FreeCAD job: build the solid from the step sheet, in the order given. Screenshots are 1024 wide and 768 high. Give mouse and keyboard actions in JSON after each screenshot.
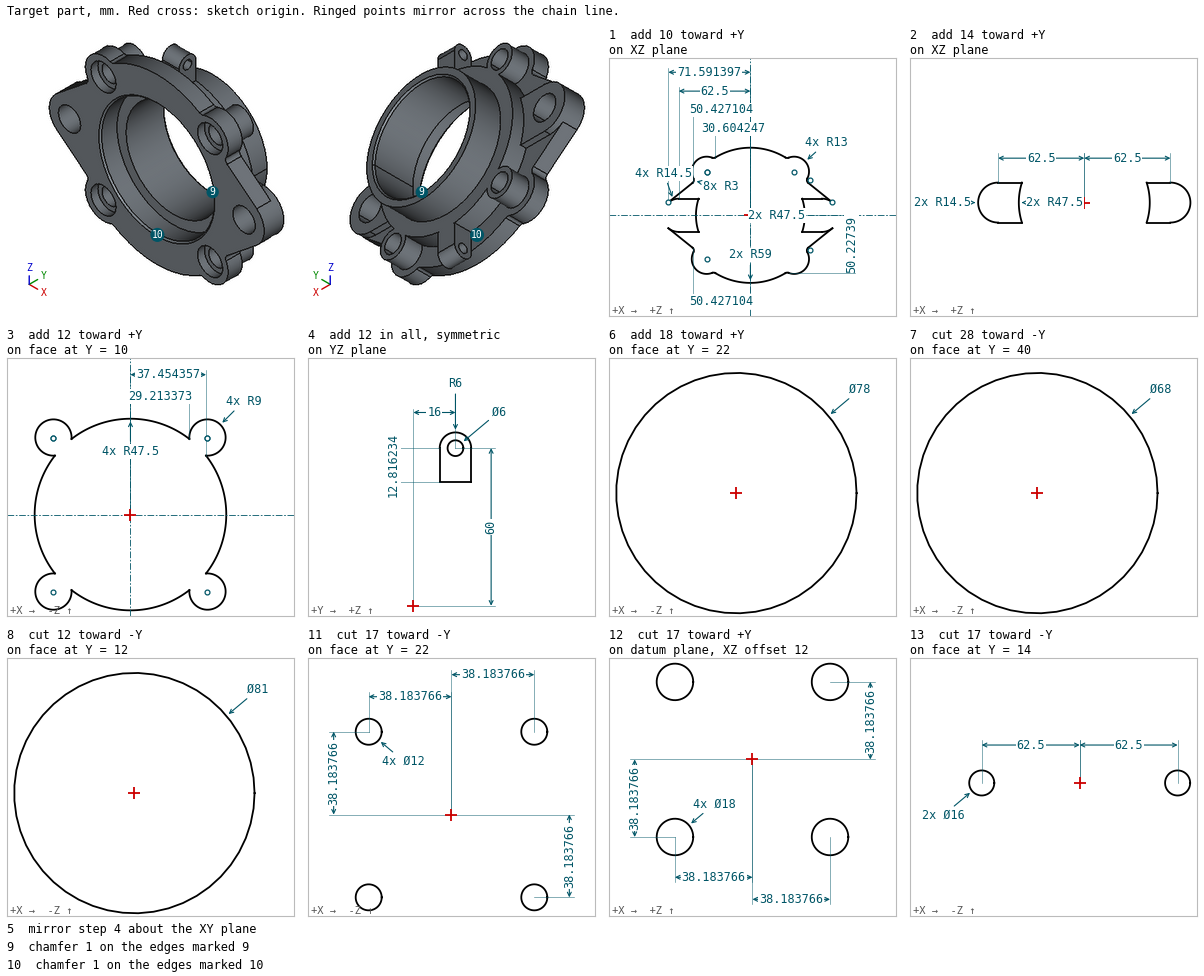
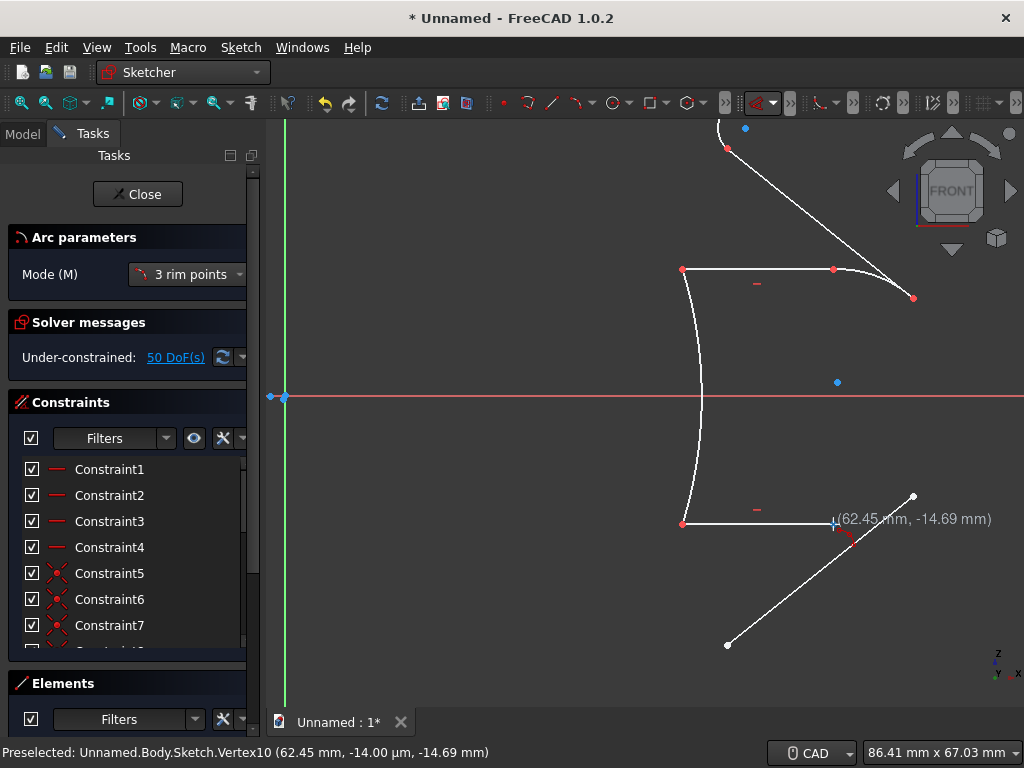
{"action": "scroll", "coordinate": [702, 421], "scroll_direction": "down", "scroll_amount": 6}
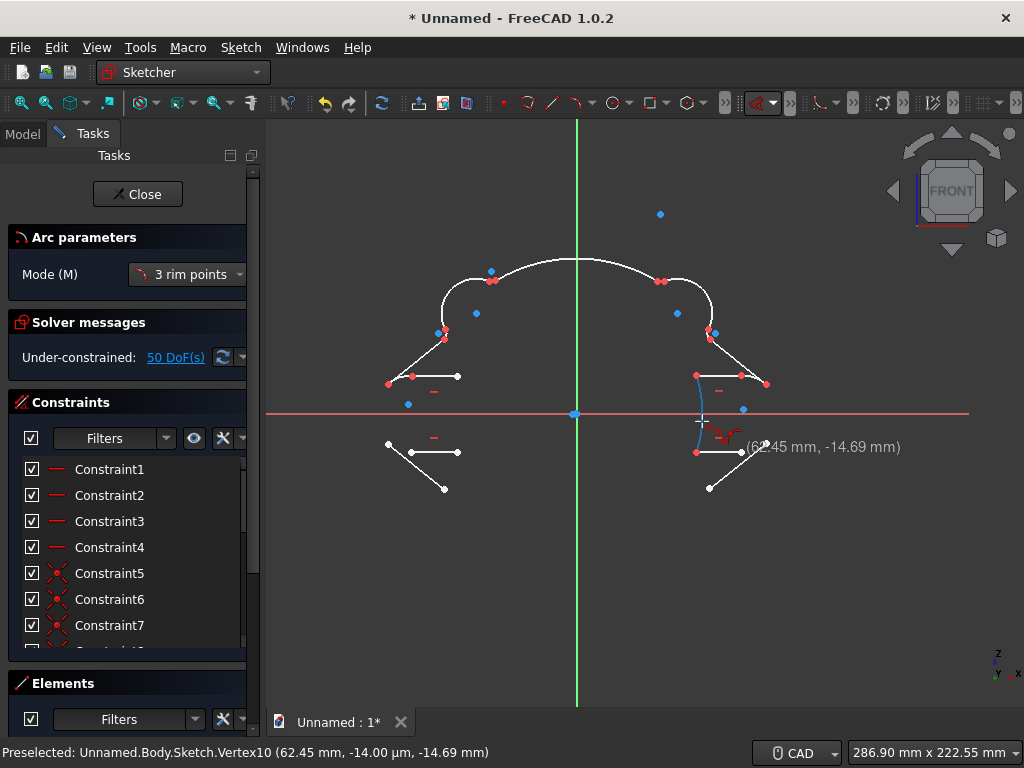
{"action": "left_click", "coordinate": [766, 444]}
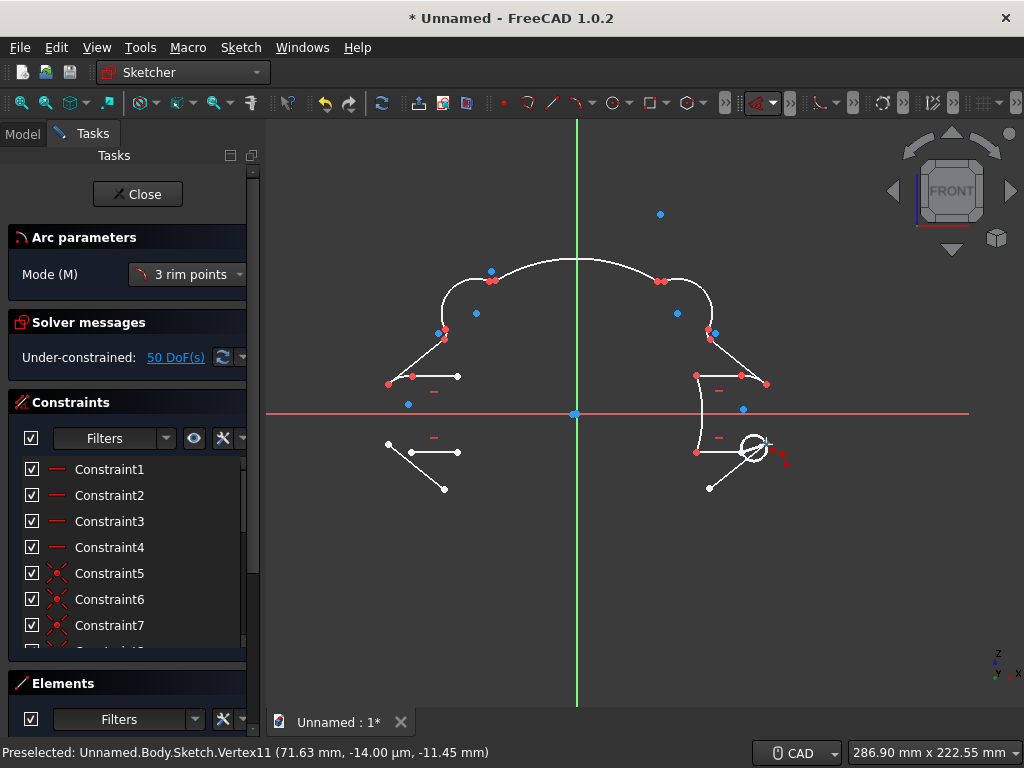
{"action": "scroll", "coordinate": [755, 450], "scroll_direction": "up", "scroll_amount": 10}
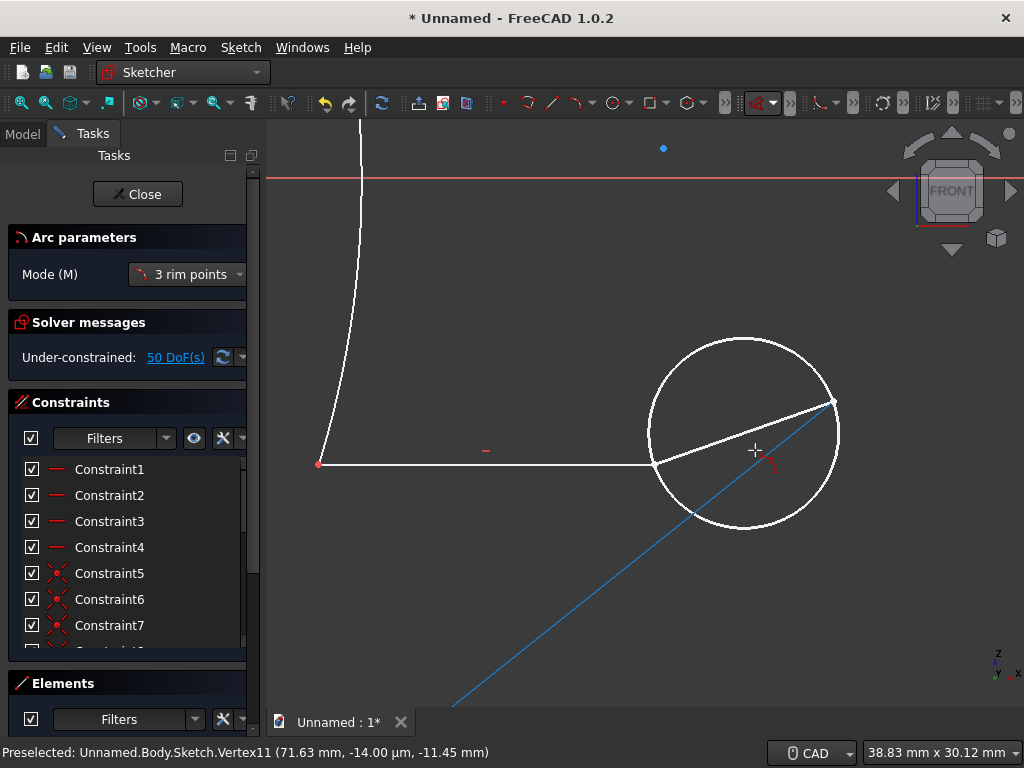
{"action": "left_click", "coordinate": [749, 445]}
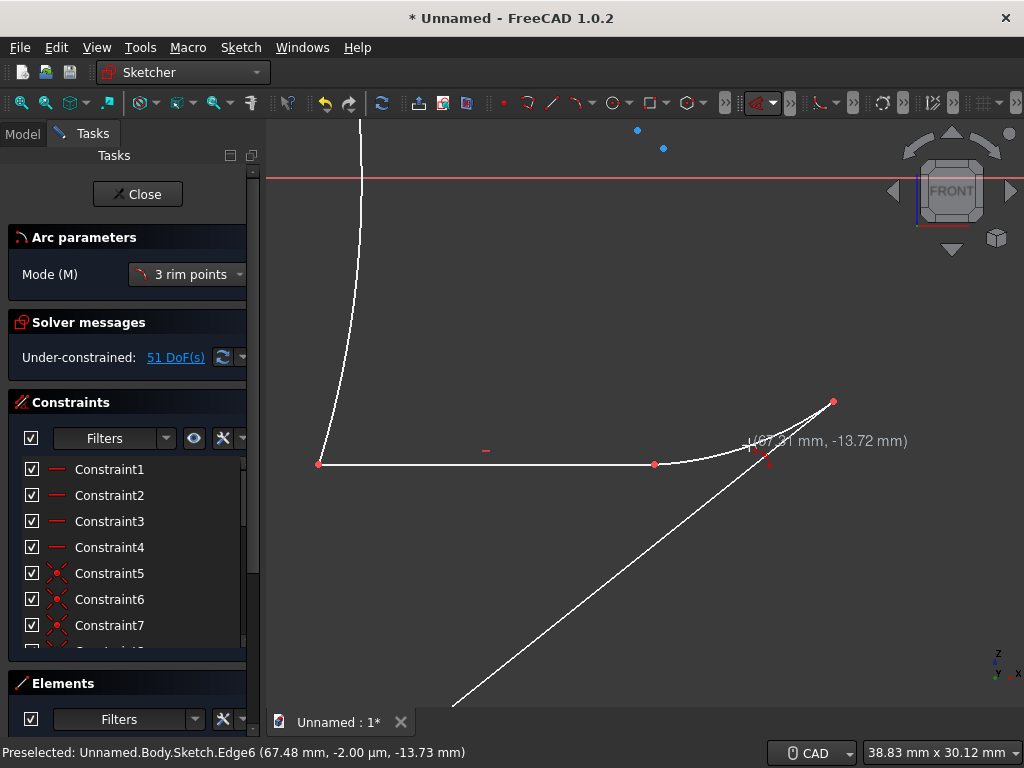
{"action": "scroll", "coordinate": [755, 450], "scroll_direction": "down", "scroll_amount": 10}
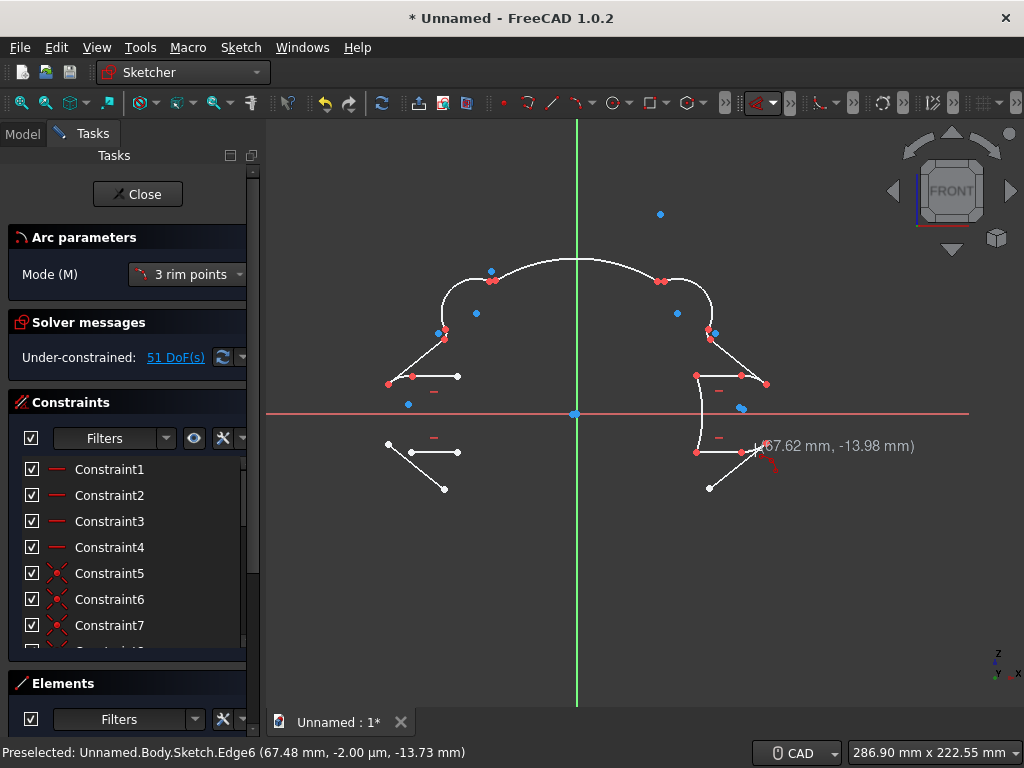
{"action": "left_click", "coordinate": [710, 489]}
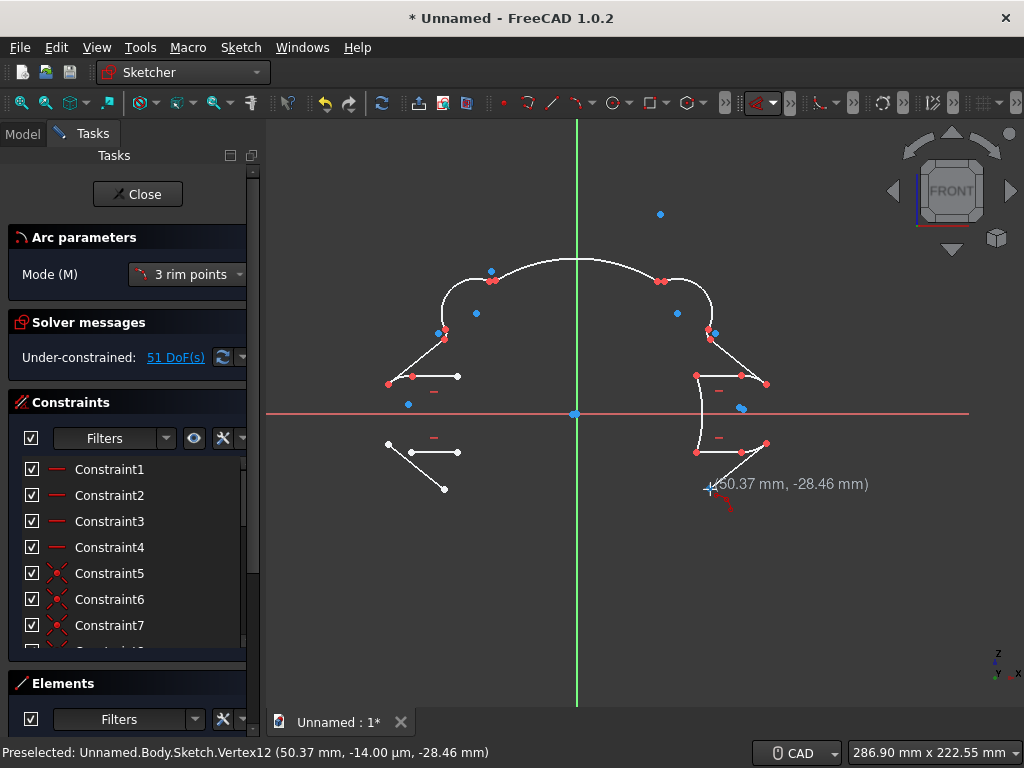
{"action": "scroll", "coordinate": [708, 498], "scroll_direction": "up", "scroll_amount": 3}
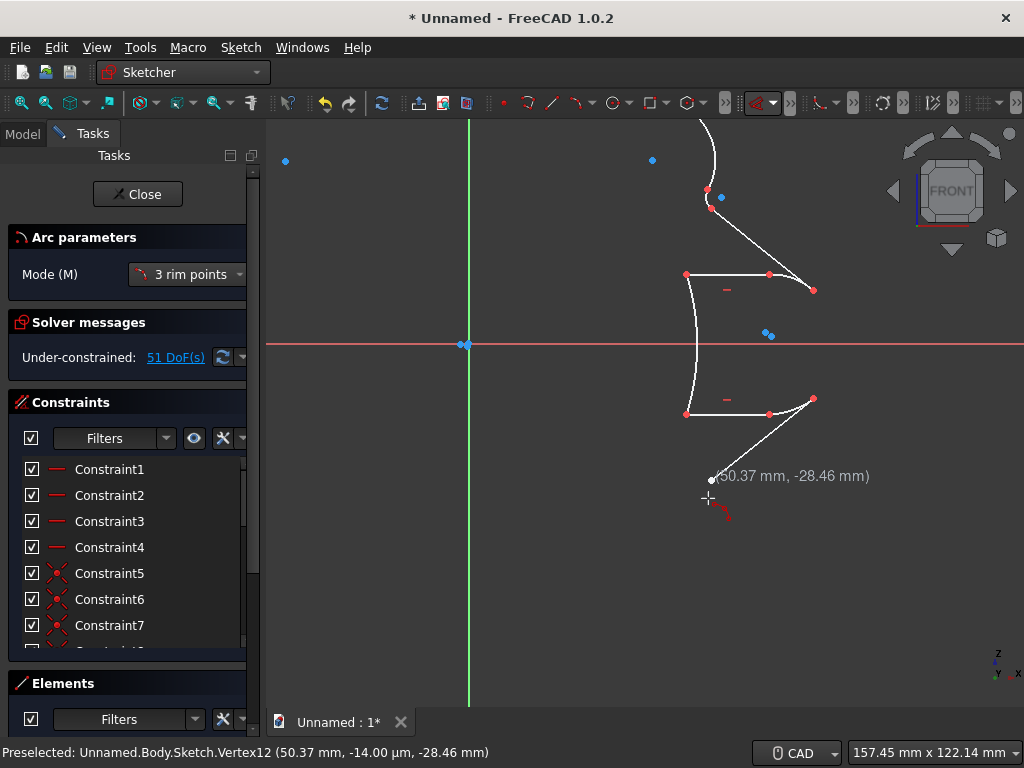
{"action": "left_click", "coordinate": [708, 498]}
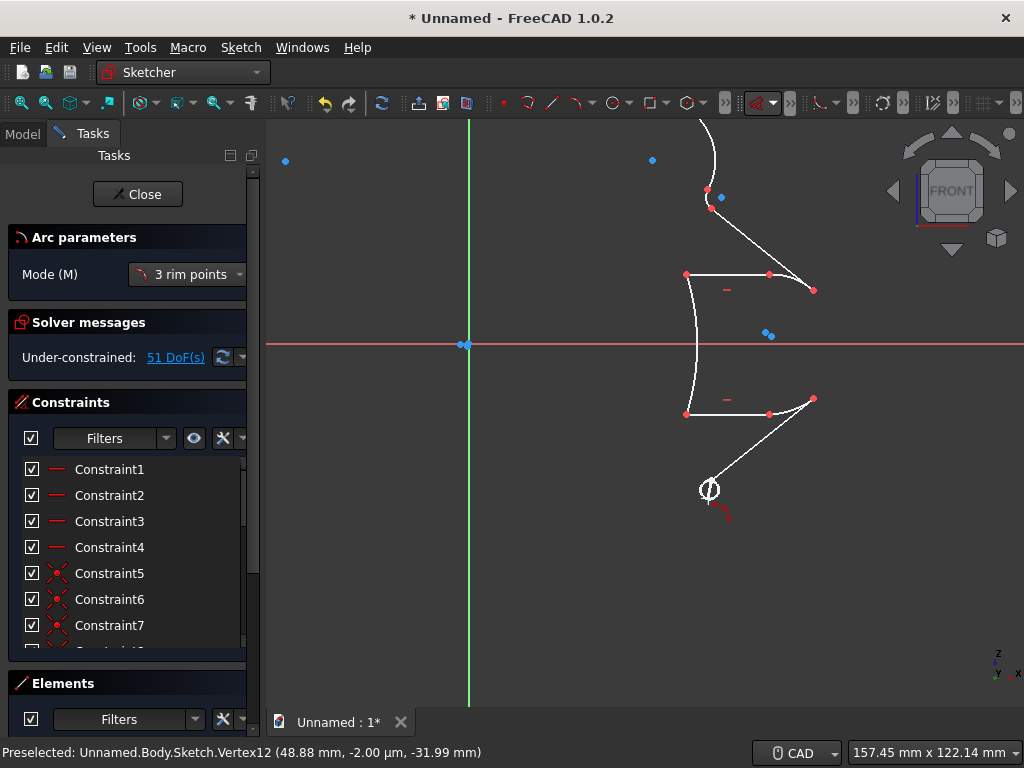
{"action": "scroll", "coordinate": [706, 489], "scroll_direction": "up", "scroll_amount": 8}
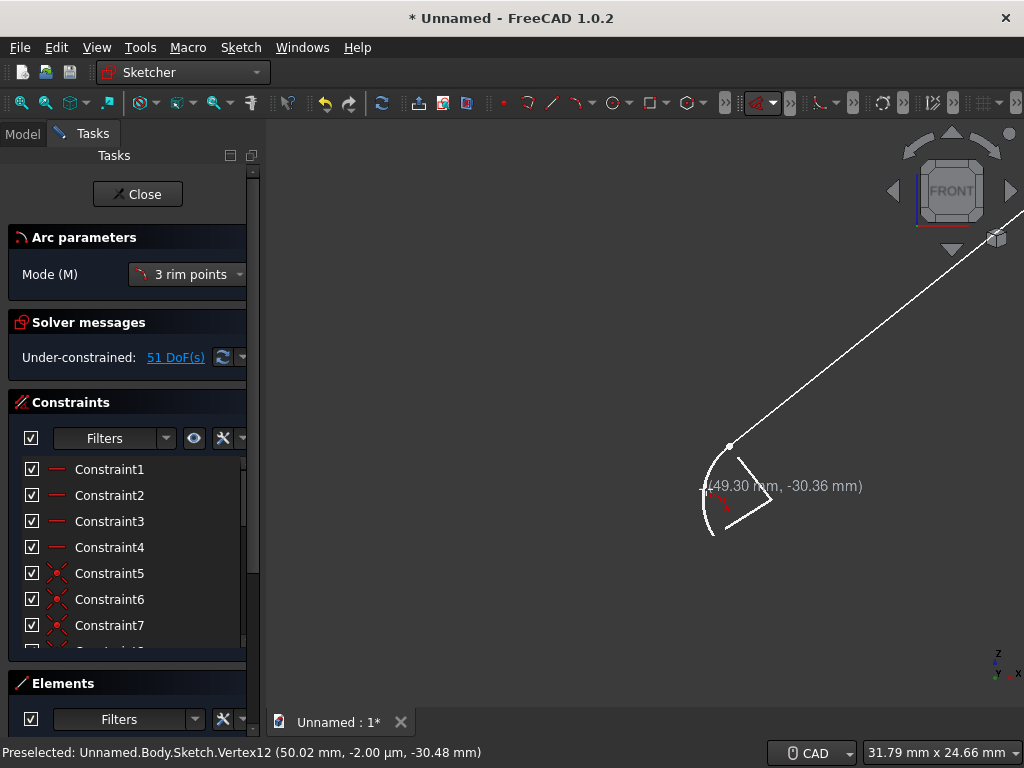
{"action": "left_click", "coordinate": [705, 484]}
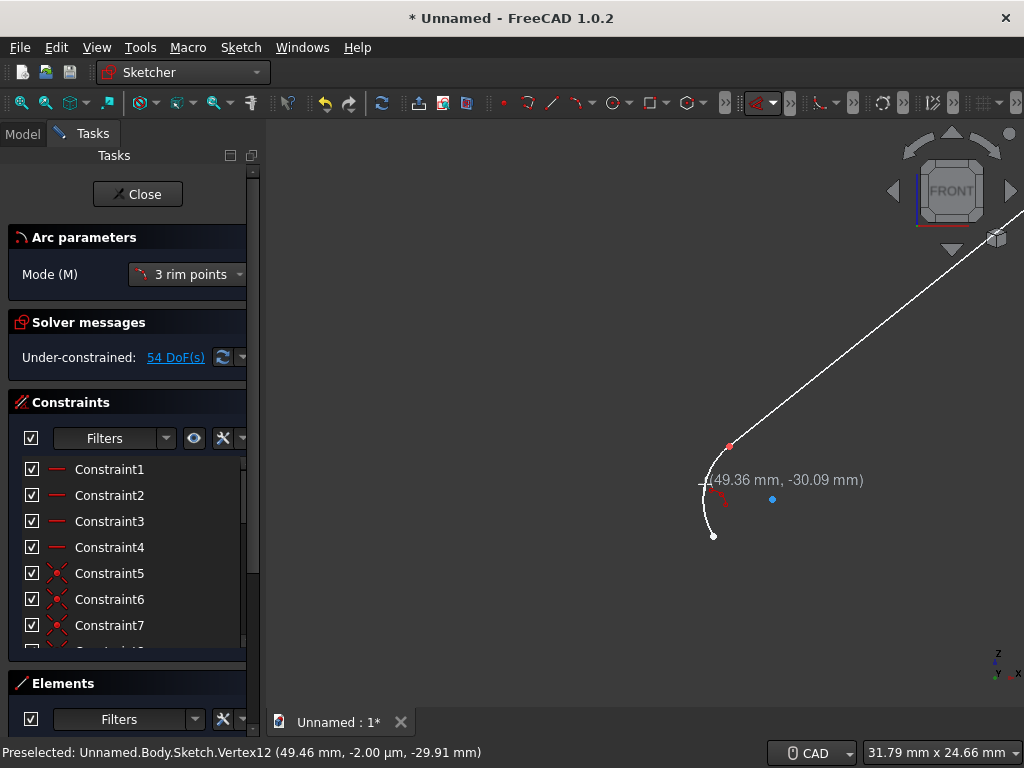
{"action": "scroll", "coordinate": [707, 493], "scroll_direction": "down", "scroll_amount": 11}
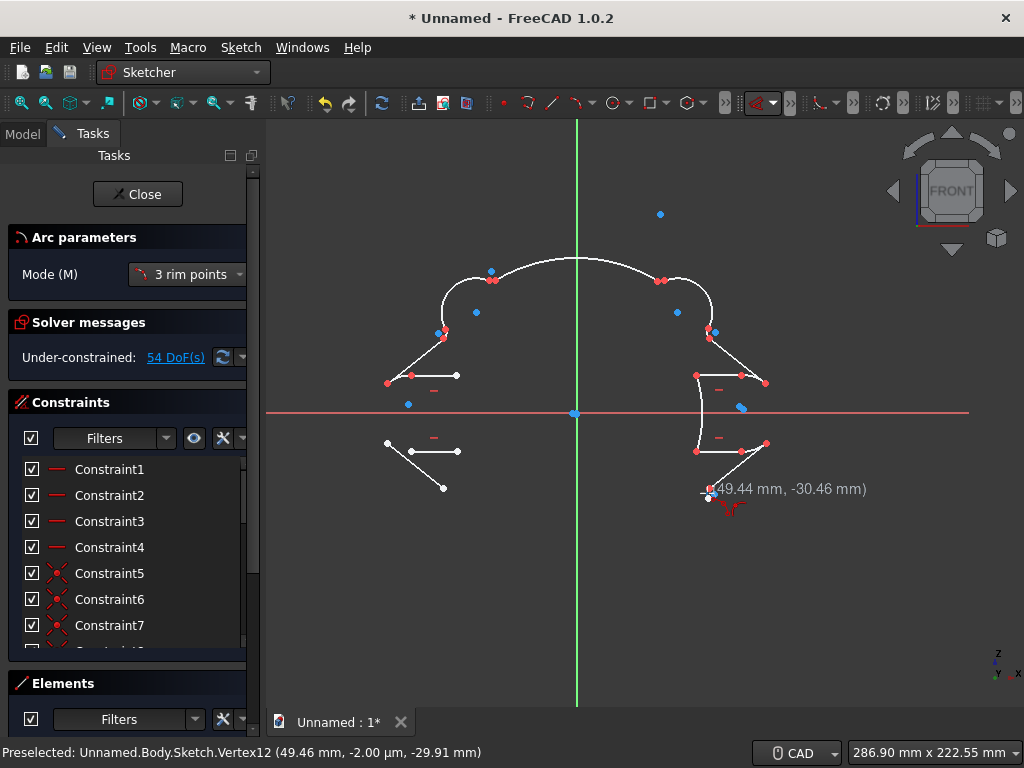
{"action": "scroll", "coordinate": [708, 498], "scroll_direction": "up", "scroll_amount": 4}